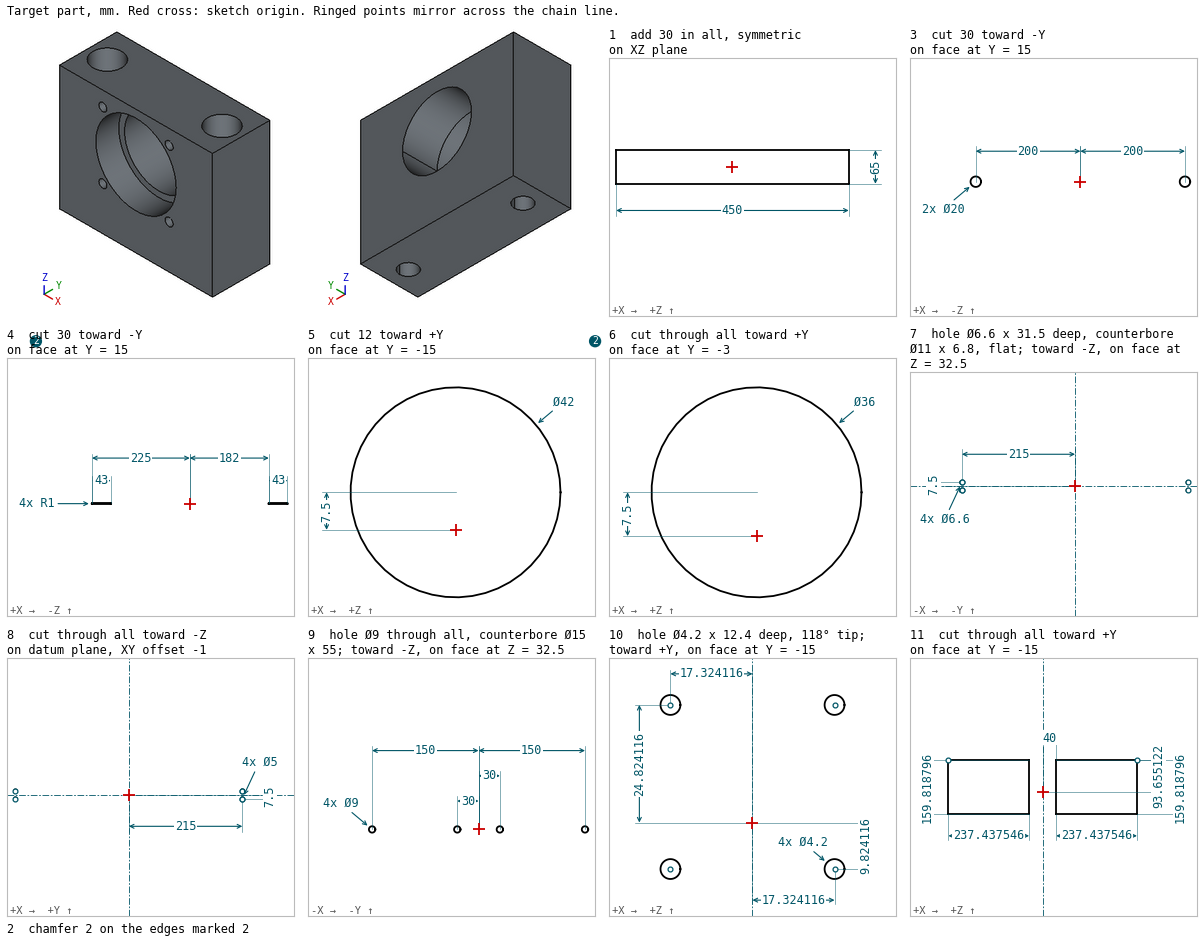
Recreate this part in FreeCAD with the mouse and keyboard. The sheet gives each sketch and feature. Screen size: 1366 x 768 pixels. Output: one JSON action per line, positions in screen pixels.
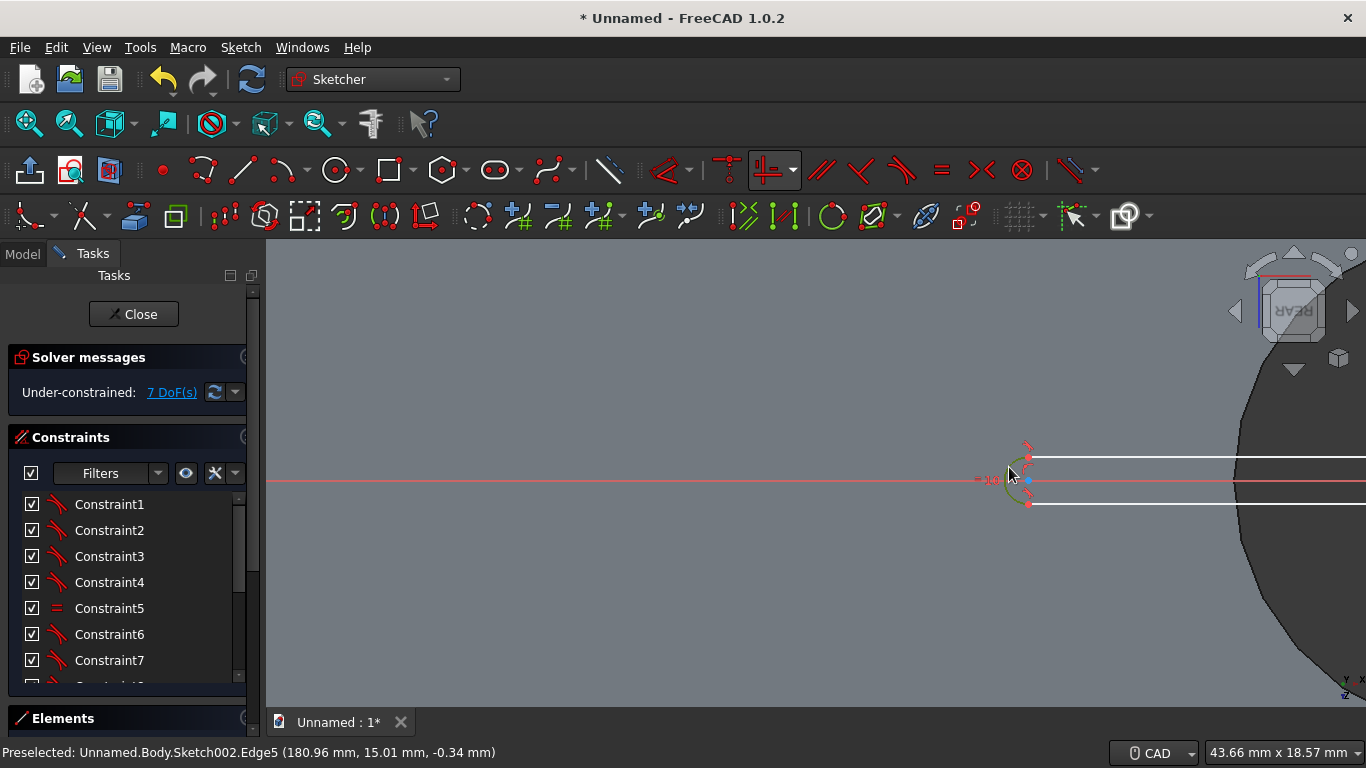
{"action": "key", "text": "e"}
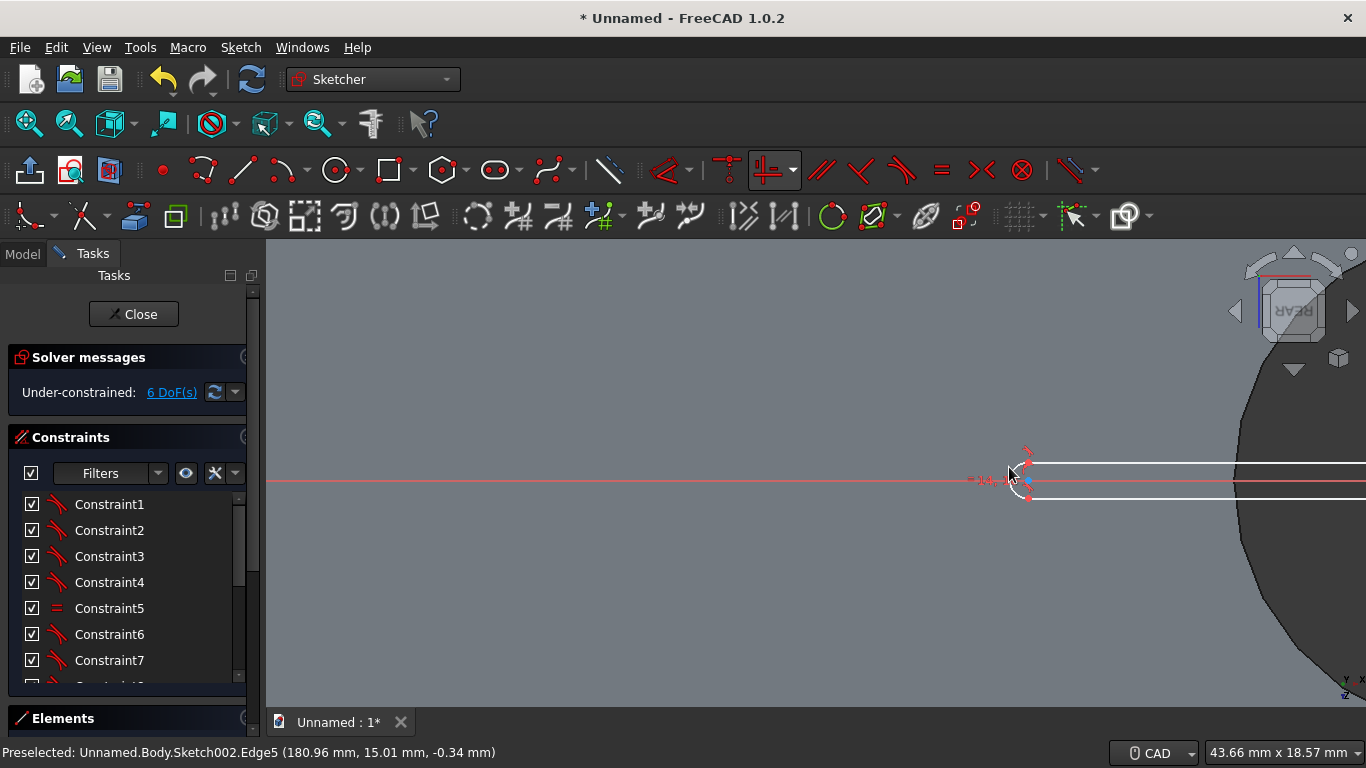
{"action": "scroll", "coordinate": [1026, 473], "scroll_direction": "down", "scroll_amount": 14}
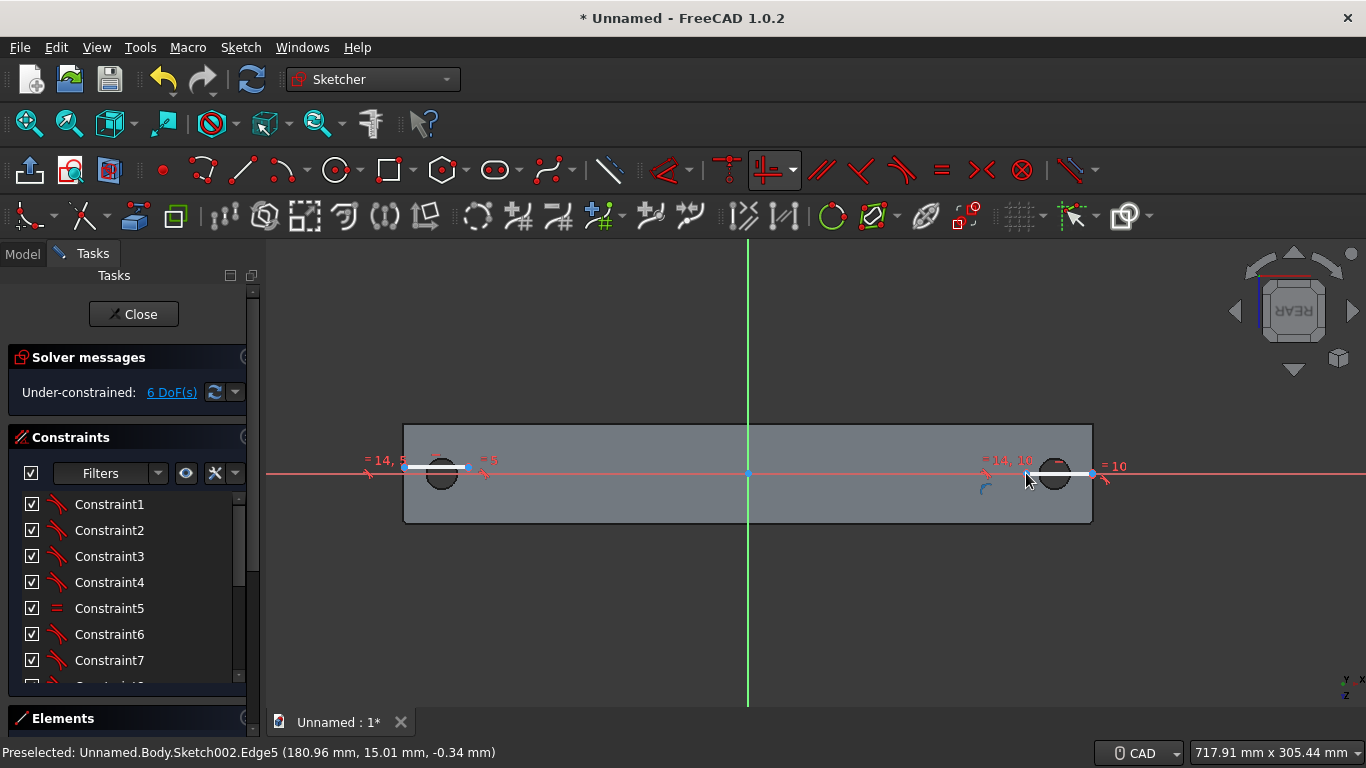
{"action": "scroll", "coordinate": [404, 467], "scroll_direction": "up", "scroll_amount": 13}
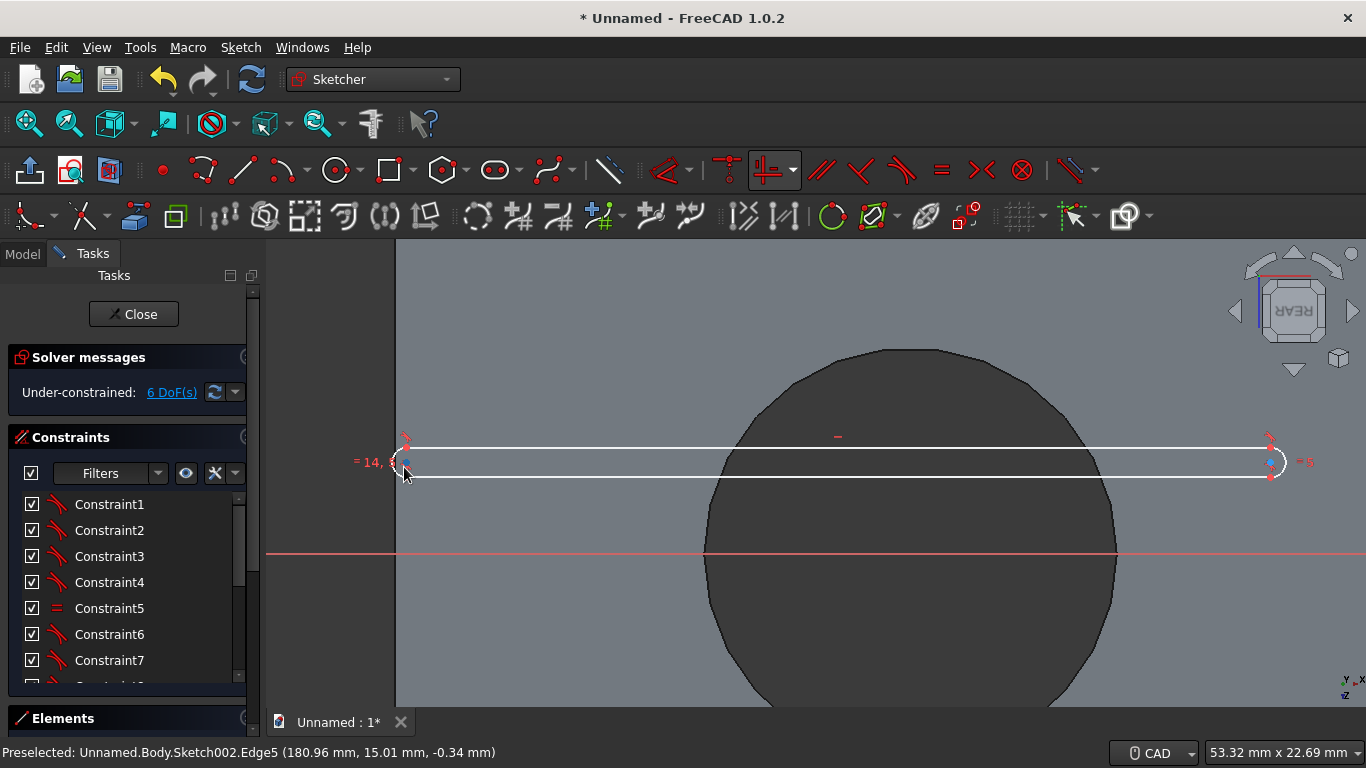
{"action": "left_click", "coordinate": [407, 463]}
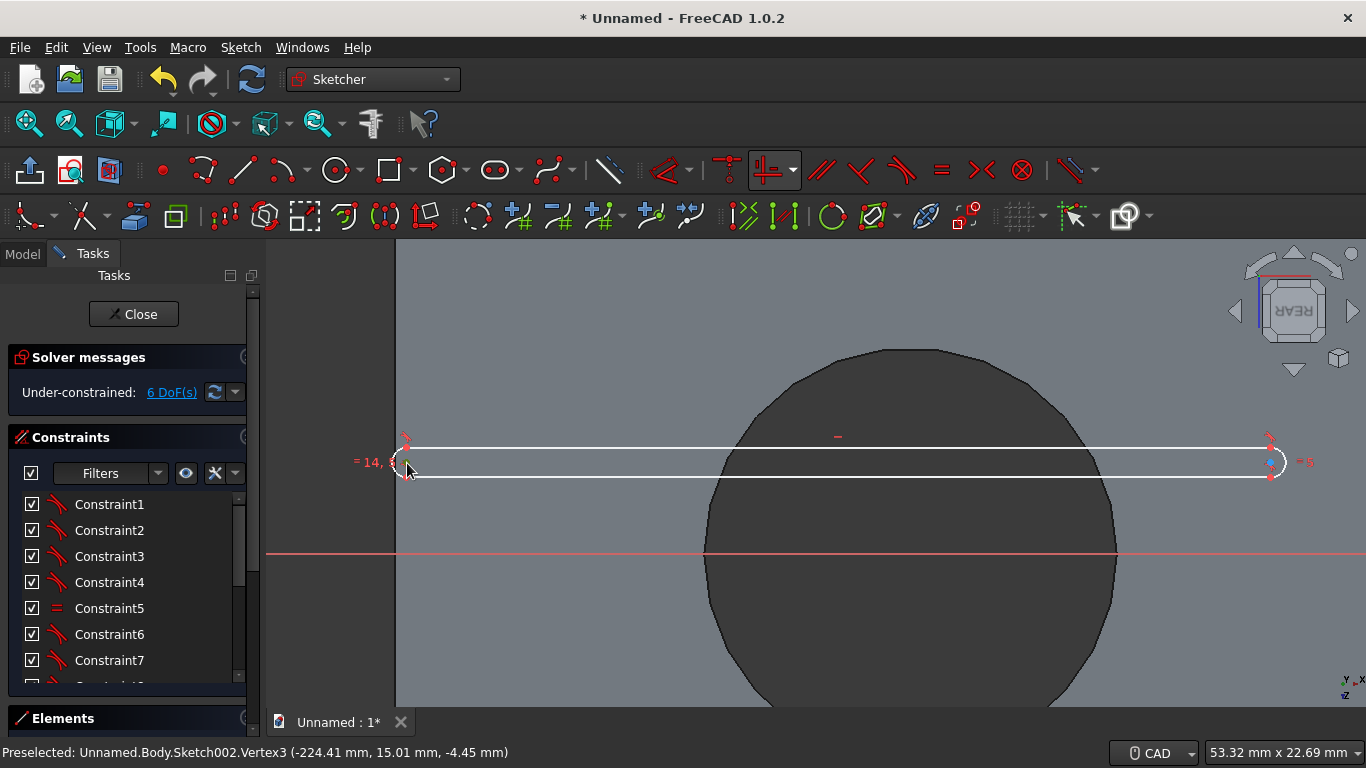
{"action": "left_click", "coordinate": [359, 554]}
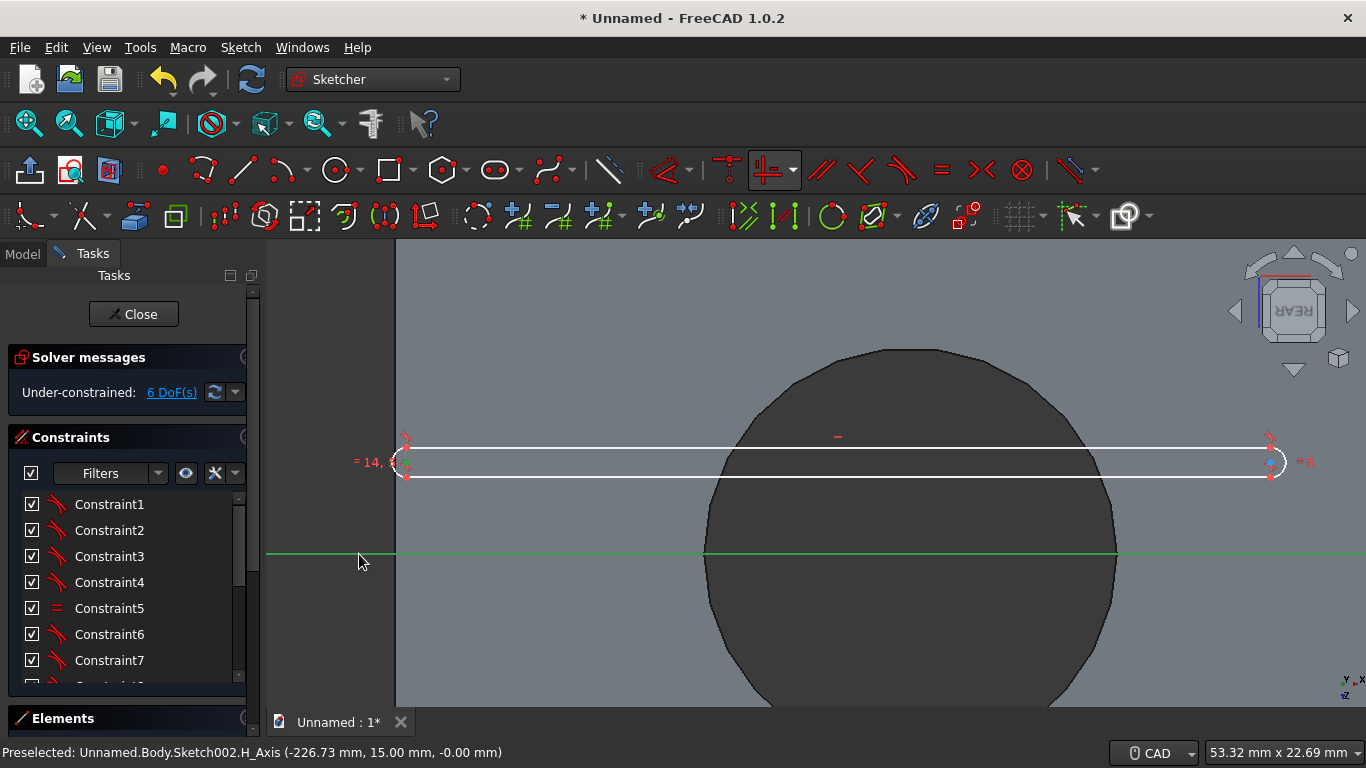
{"action": "key", "text": "c"}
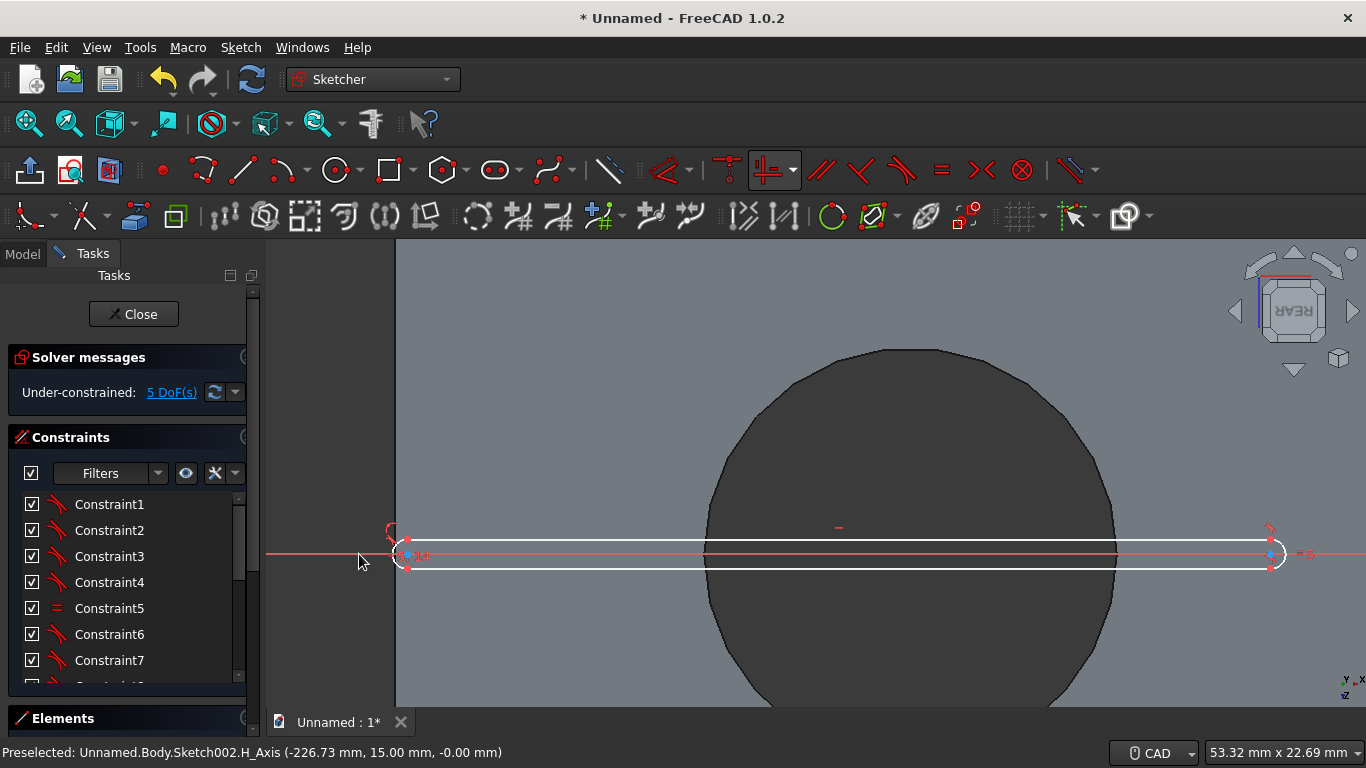
{"action": "key", "text": "d"}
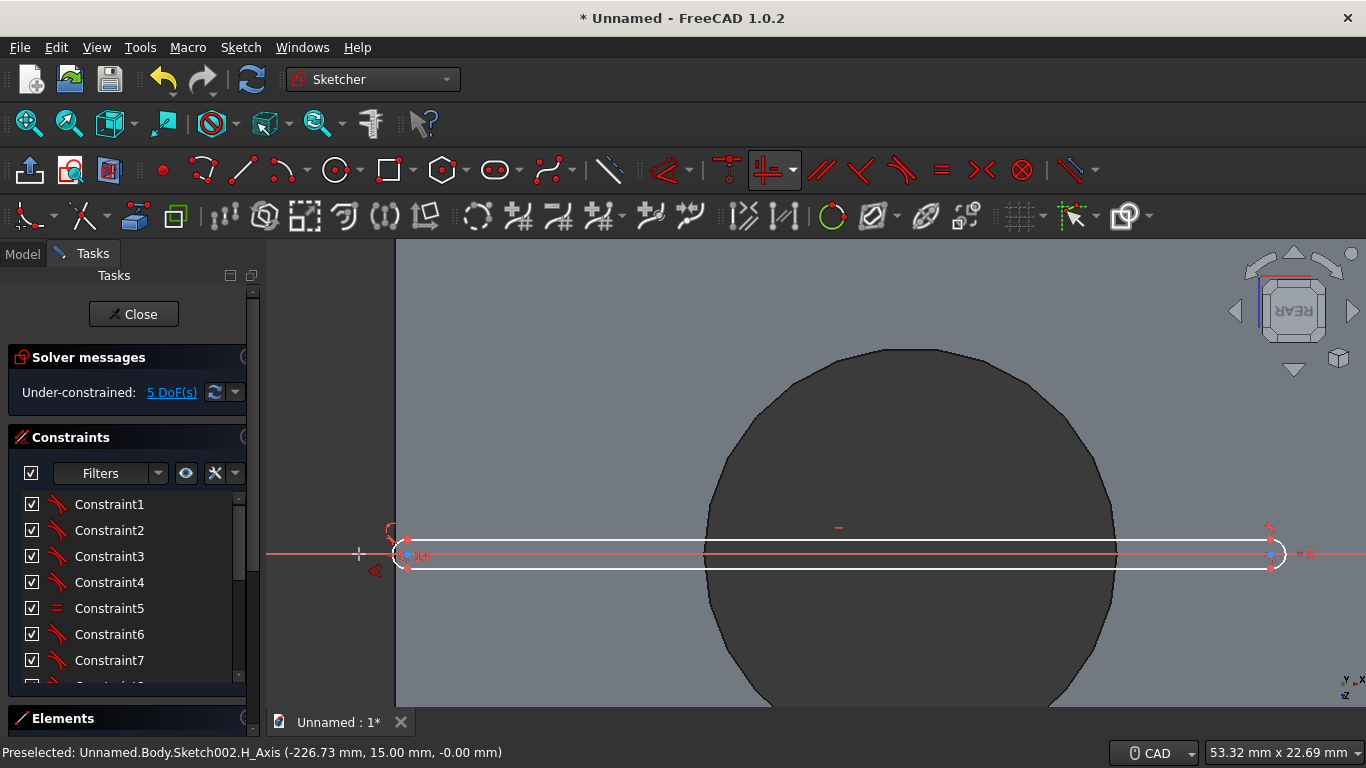
{"action": "scroll", "coordinate": [393, 554], "scroll_direction": "up", "scroll_amount": 4}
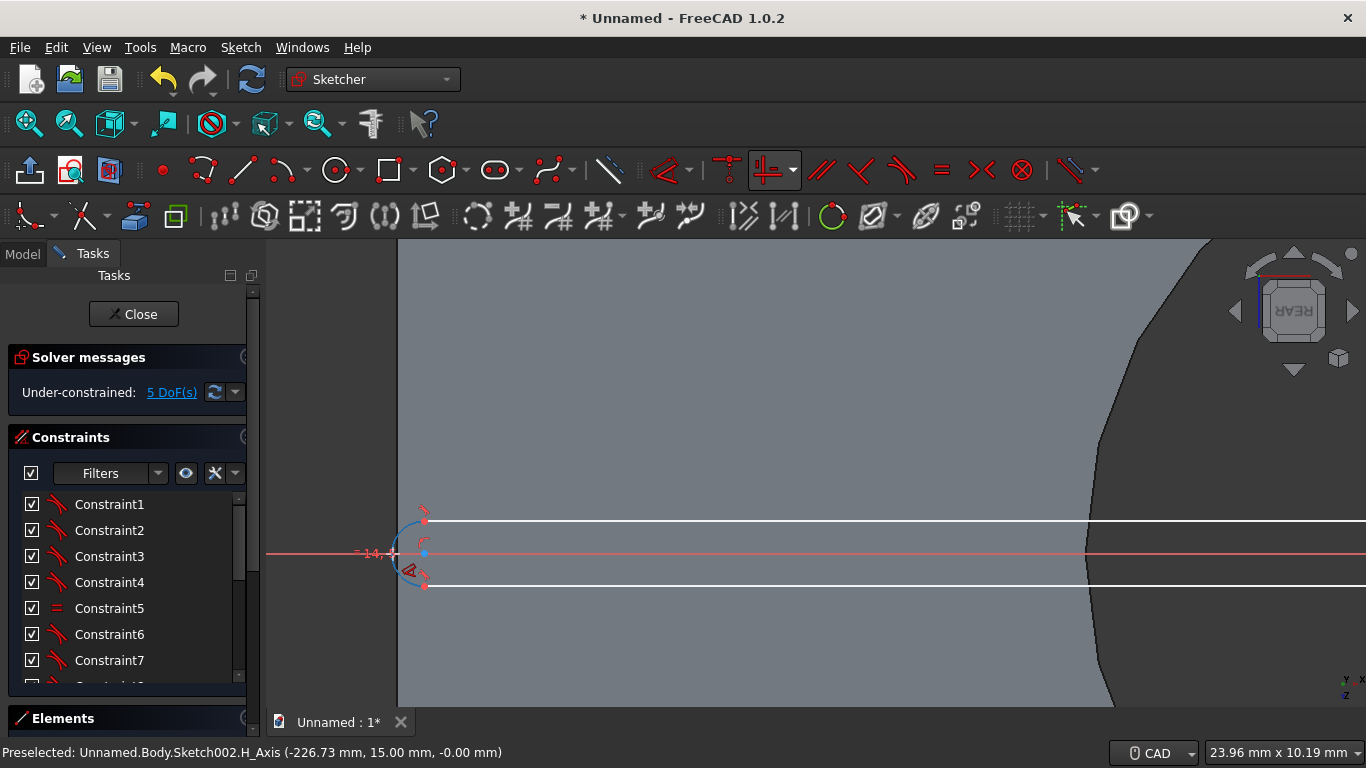
{"action": "left_click", "coordinate": [392, 554]}
{"action": "left_click", "coordinate": [368, 523]}